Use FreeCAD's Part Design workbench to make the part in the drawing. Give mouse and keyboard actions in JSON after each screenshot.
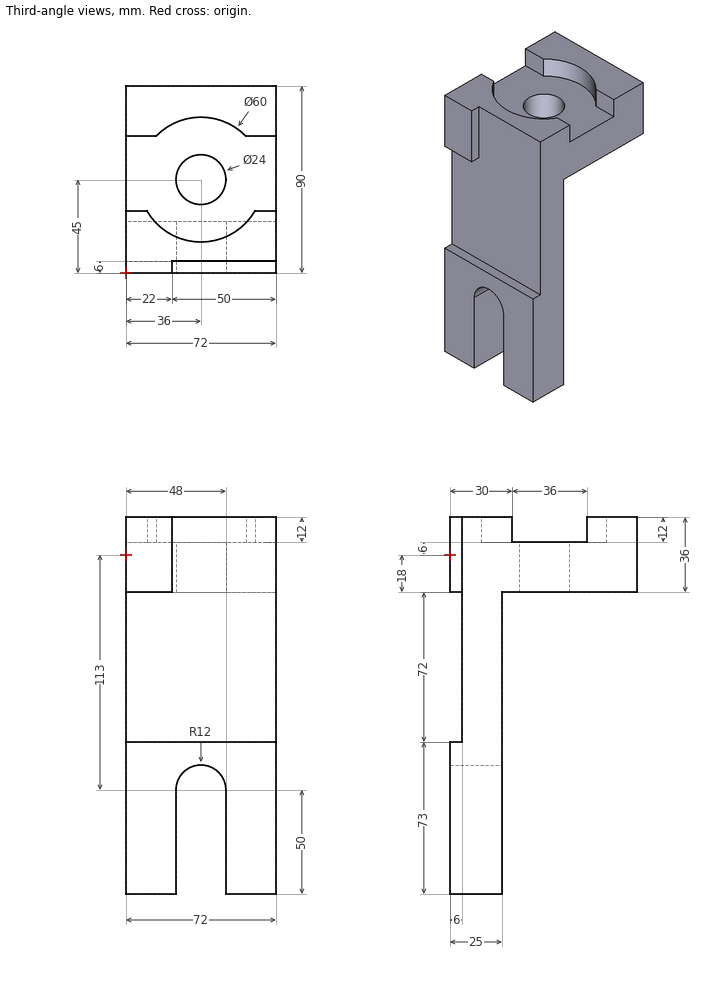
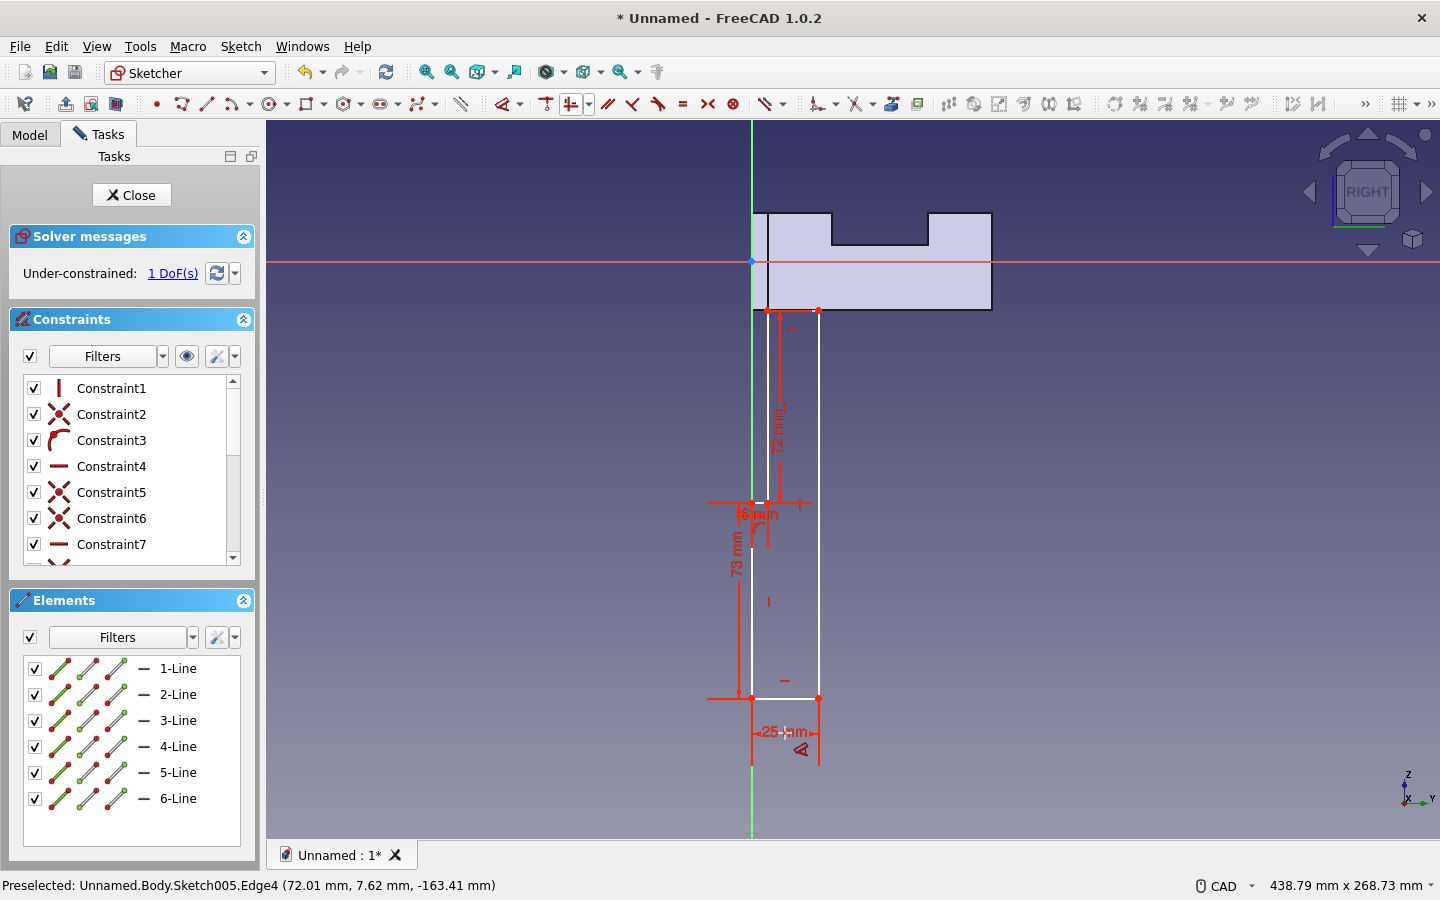
{"action": "left_click", "coordinate": [768, 311]}
{"action": "left_click", "coordinate": [718, 286]}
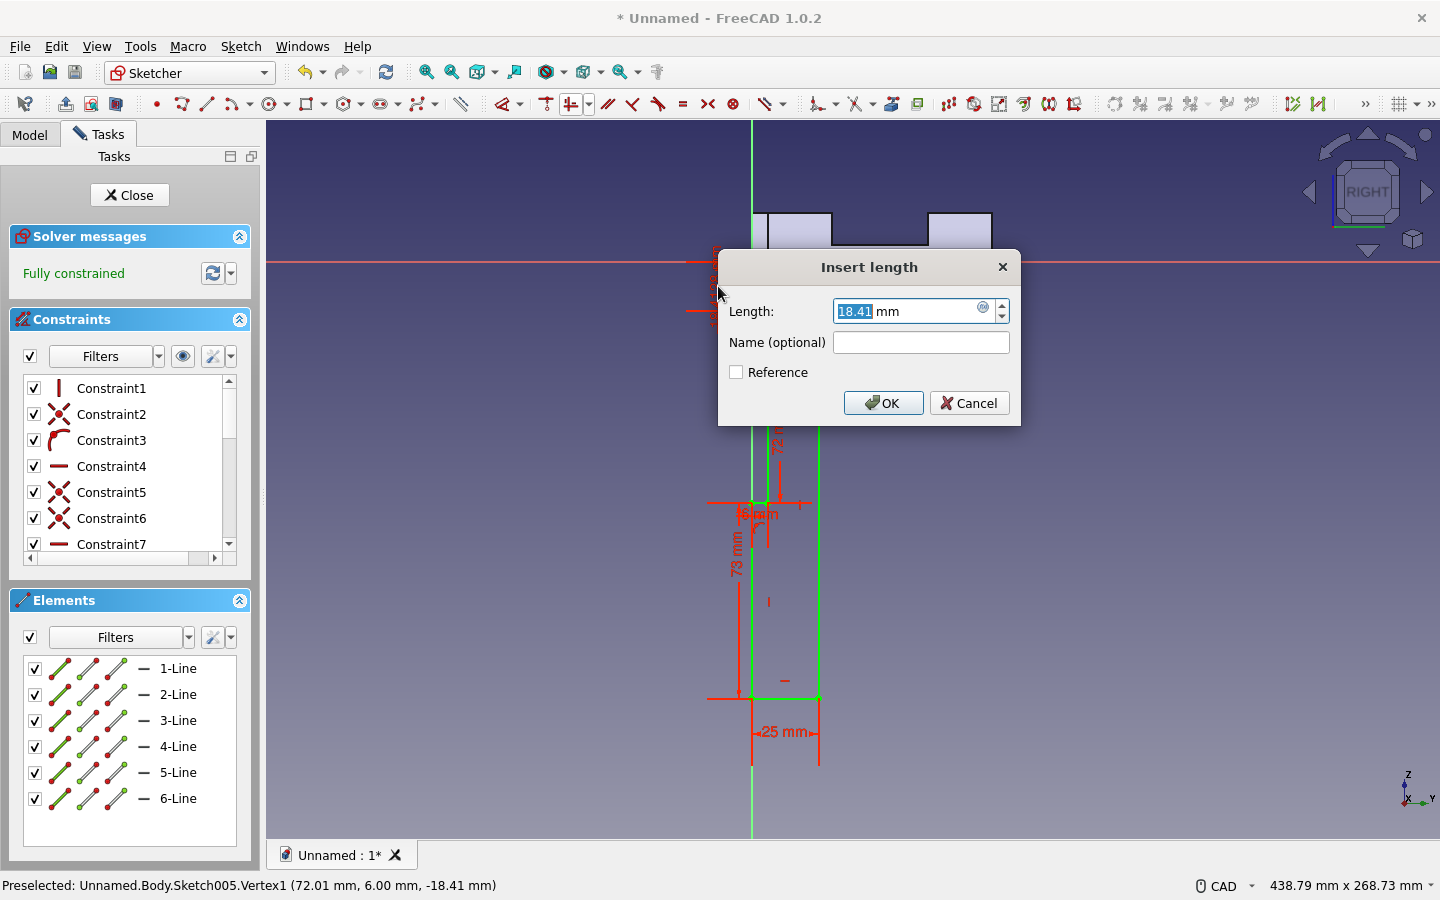
{"action": "type", "text": "18"}
{"action": "key", "text": "Return"}
{"action": "key", "text": "Escape"}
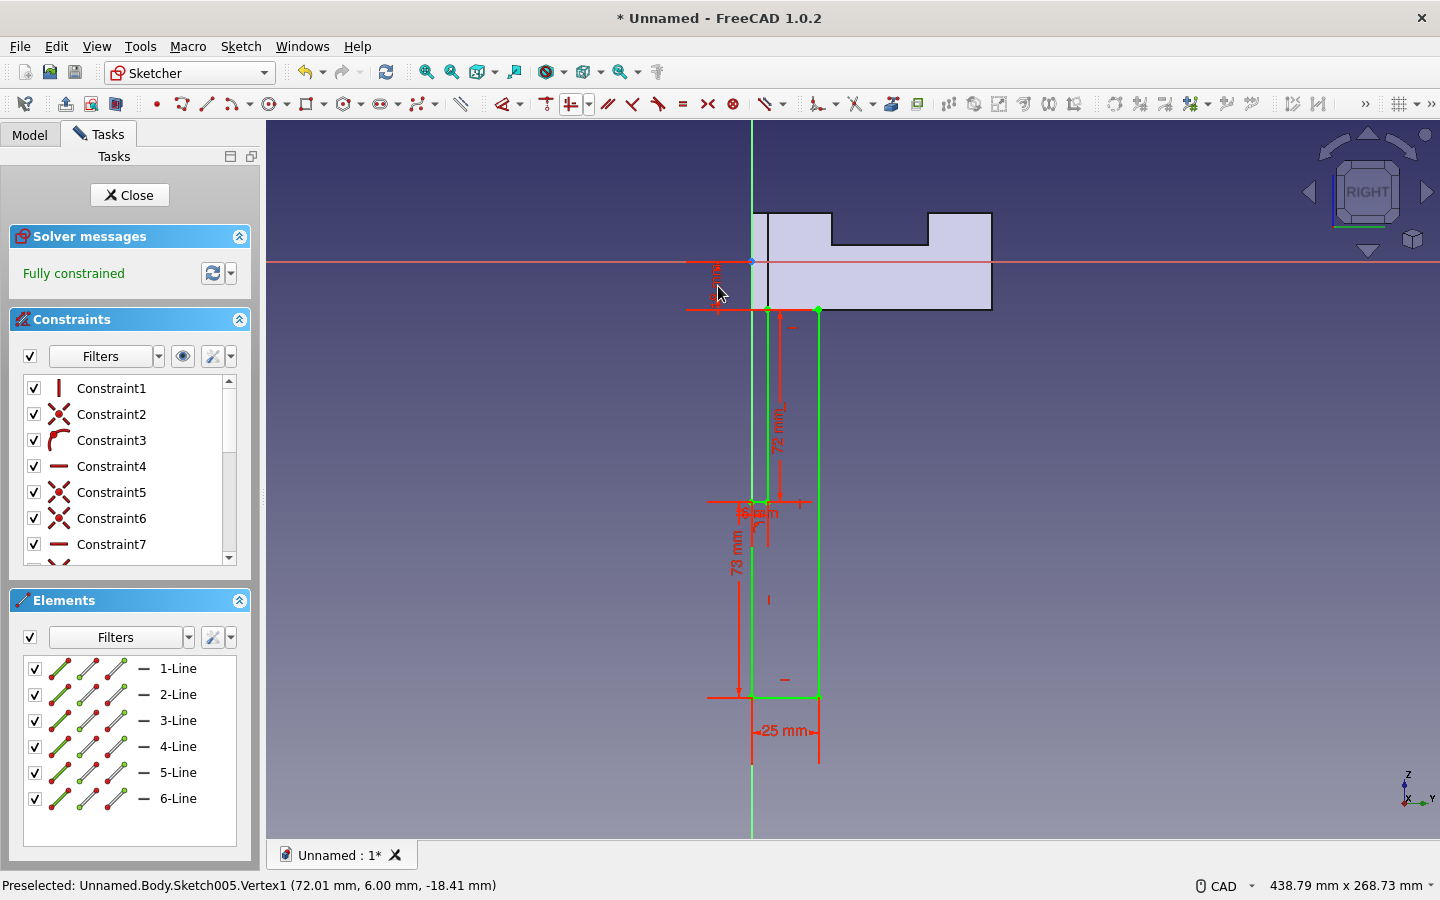
{"action": "left_click", "coordinate": [130, 195]}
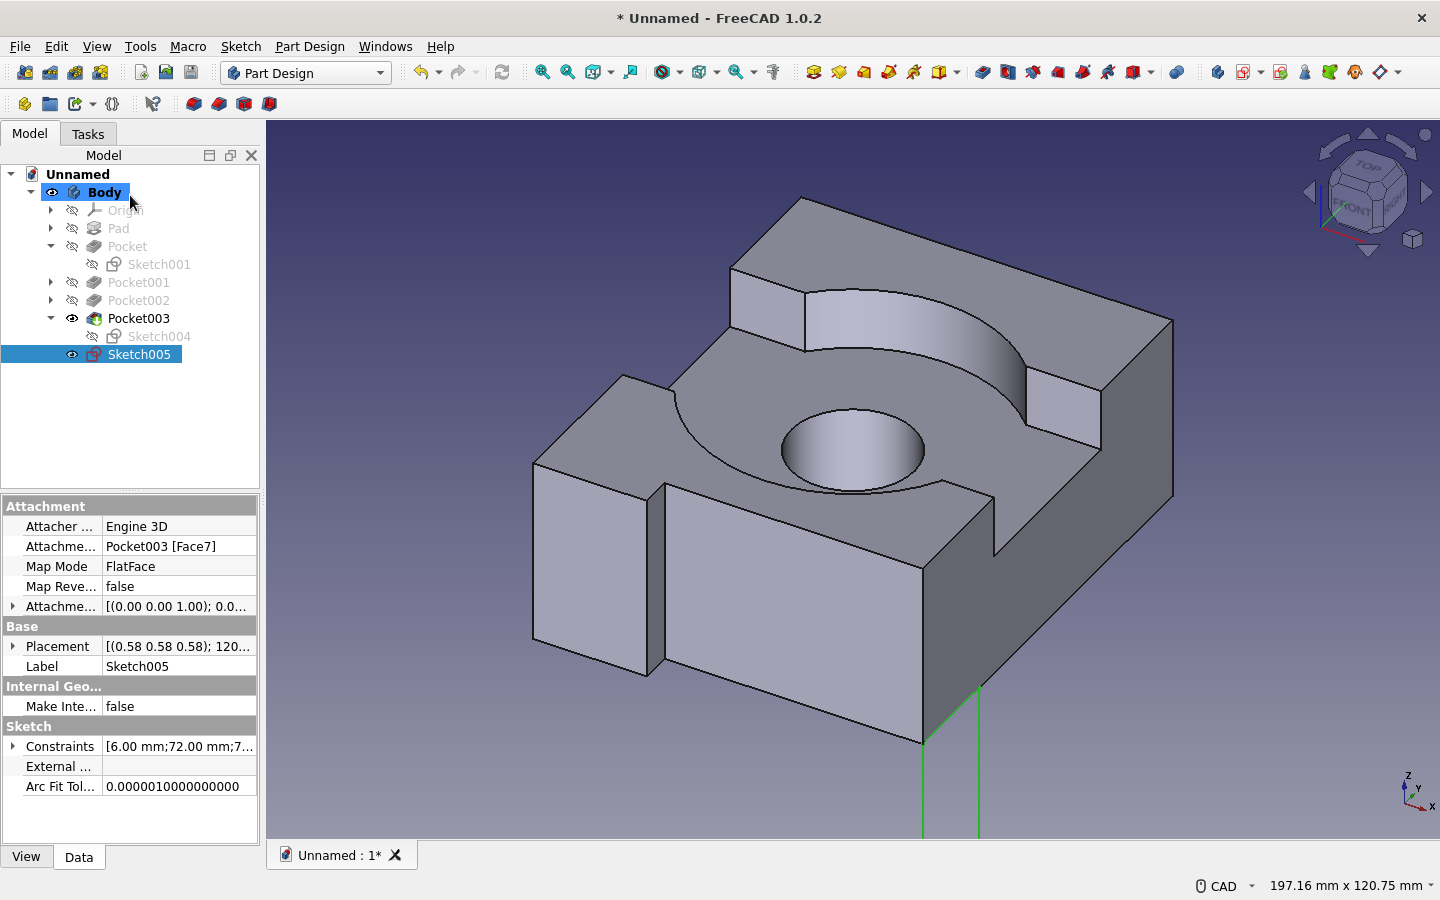
{"action": "left_click", "coordinate": [814, 72]}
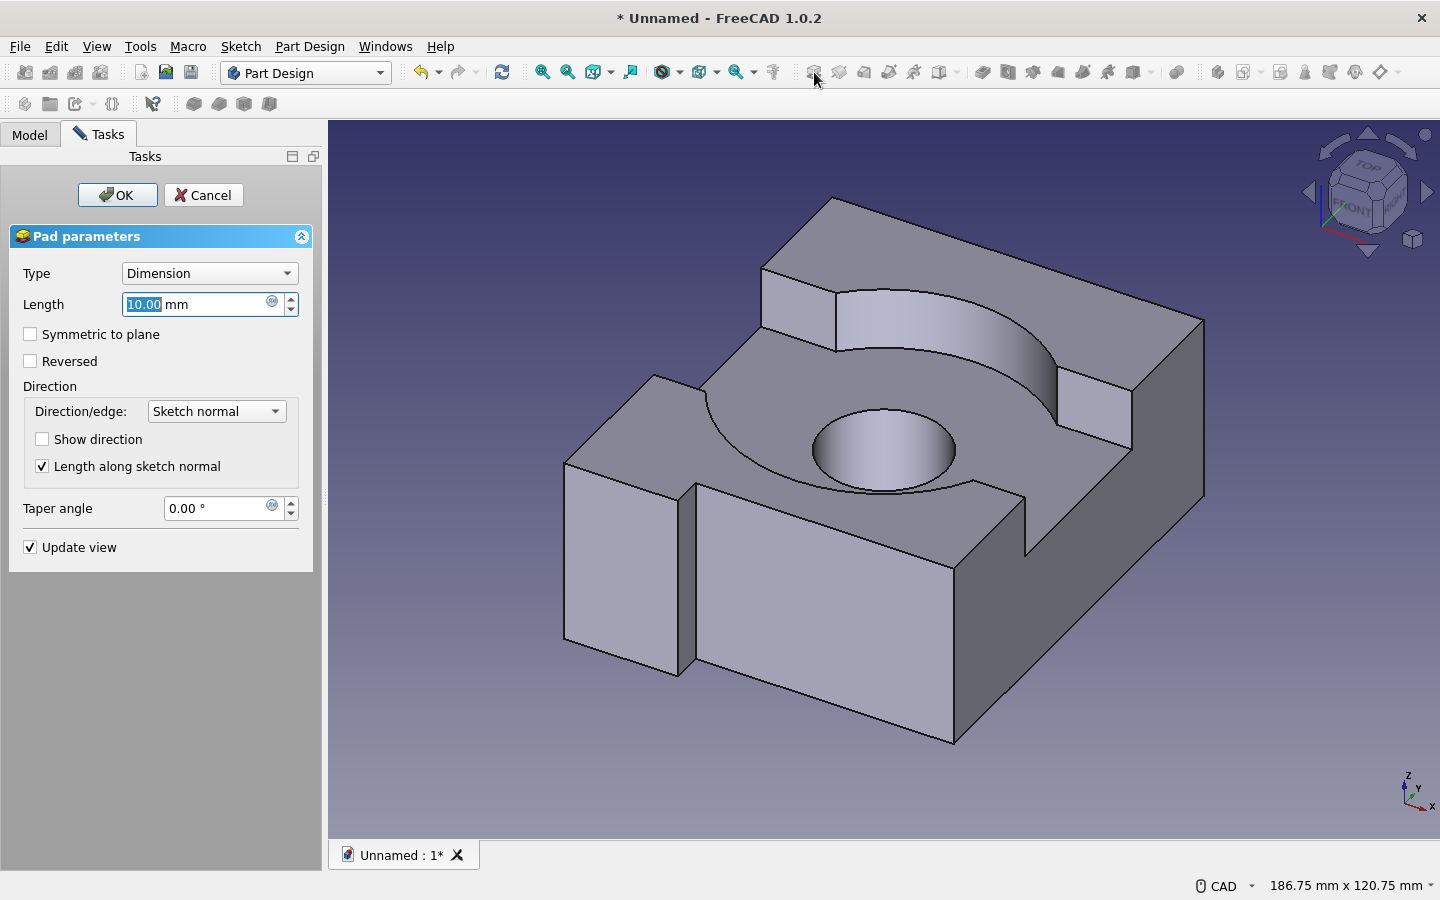
{"action": "type", "text": "72"}
{"action": "key", "text": "Tab"}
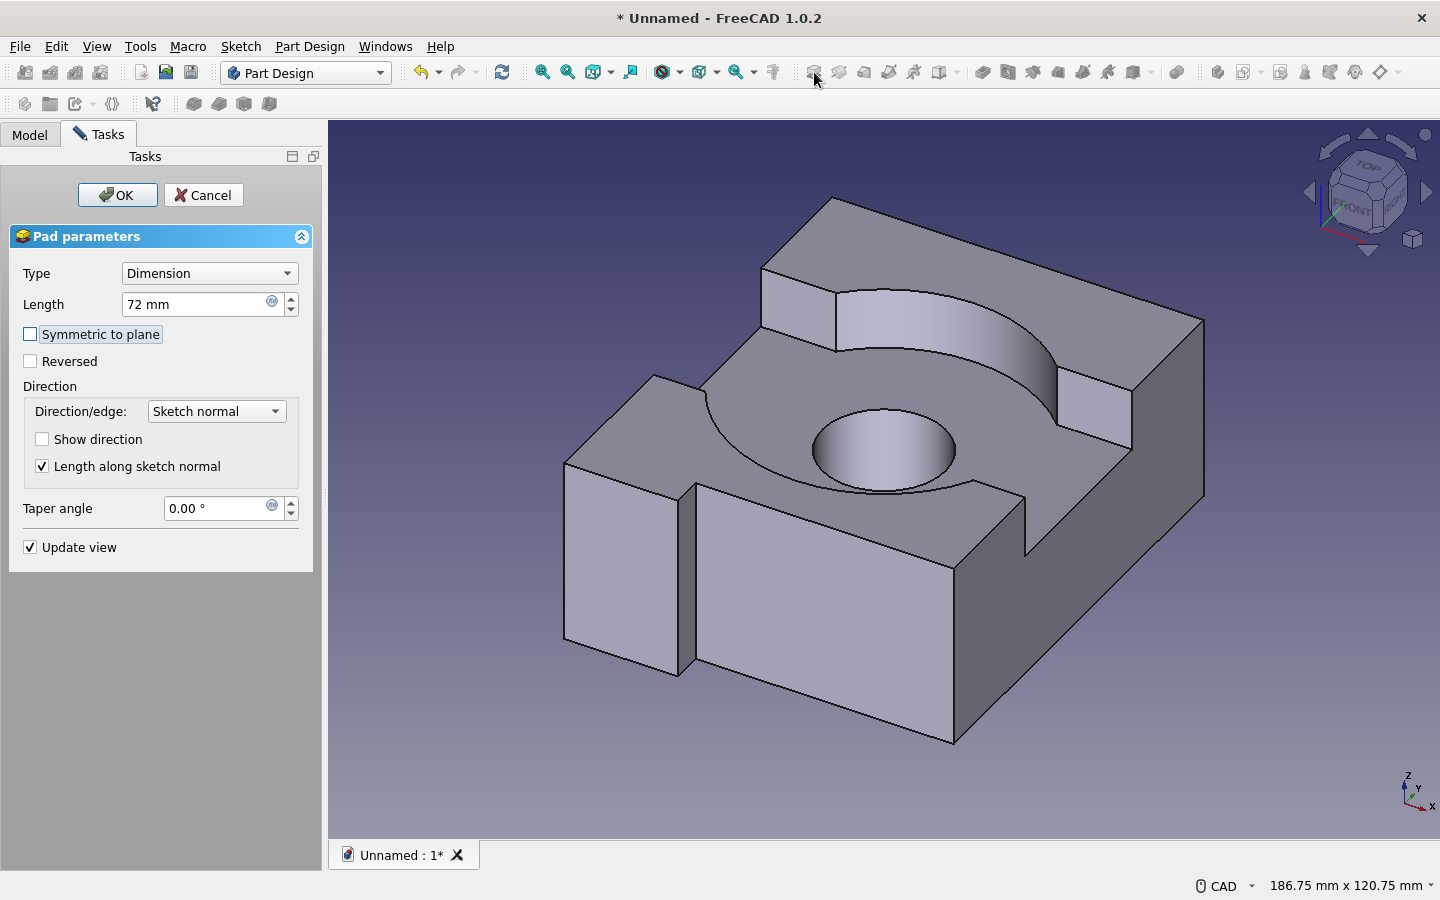
{"action": "left_click", "coordinate": [31, 361]}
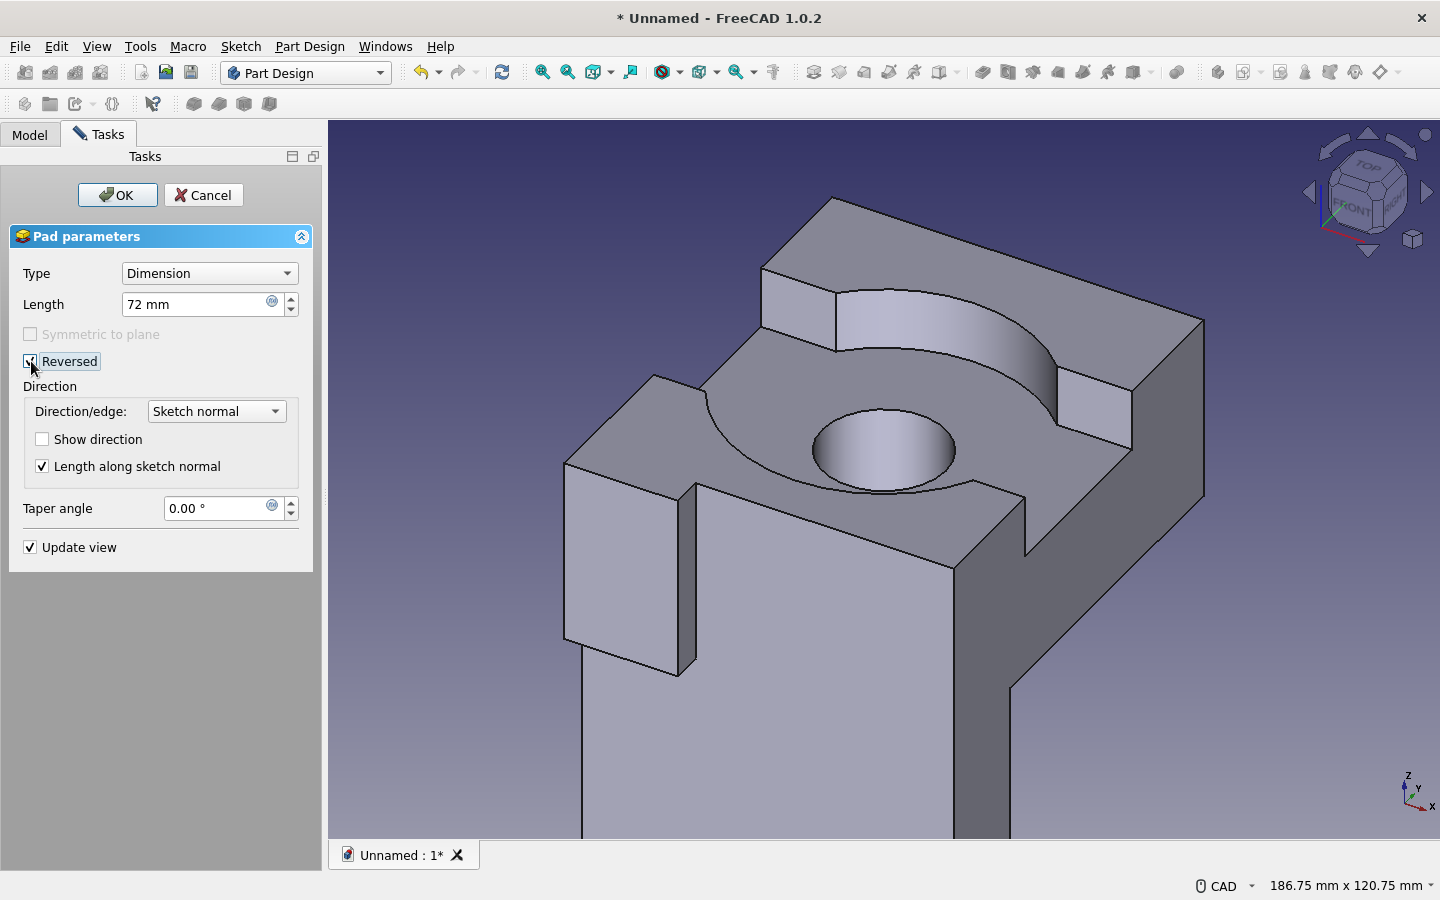
{"action": "left_click", "coordinate": [118, 195]}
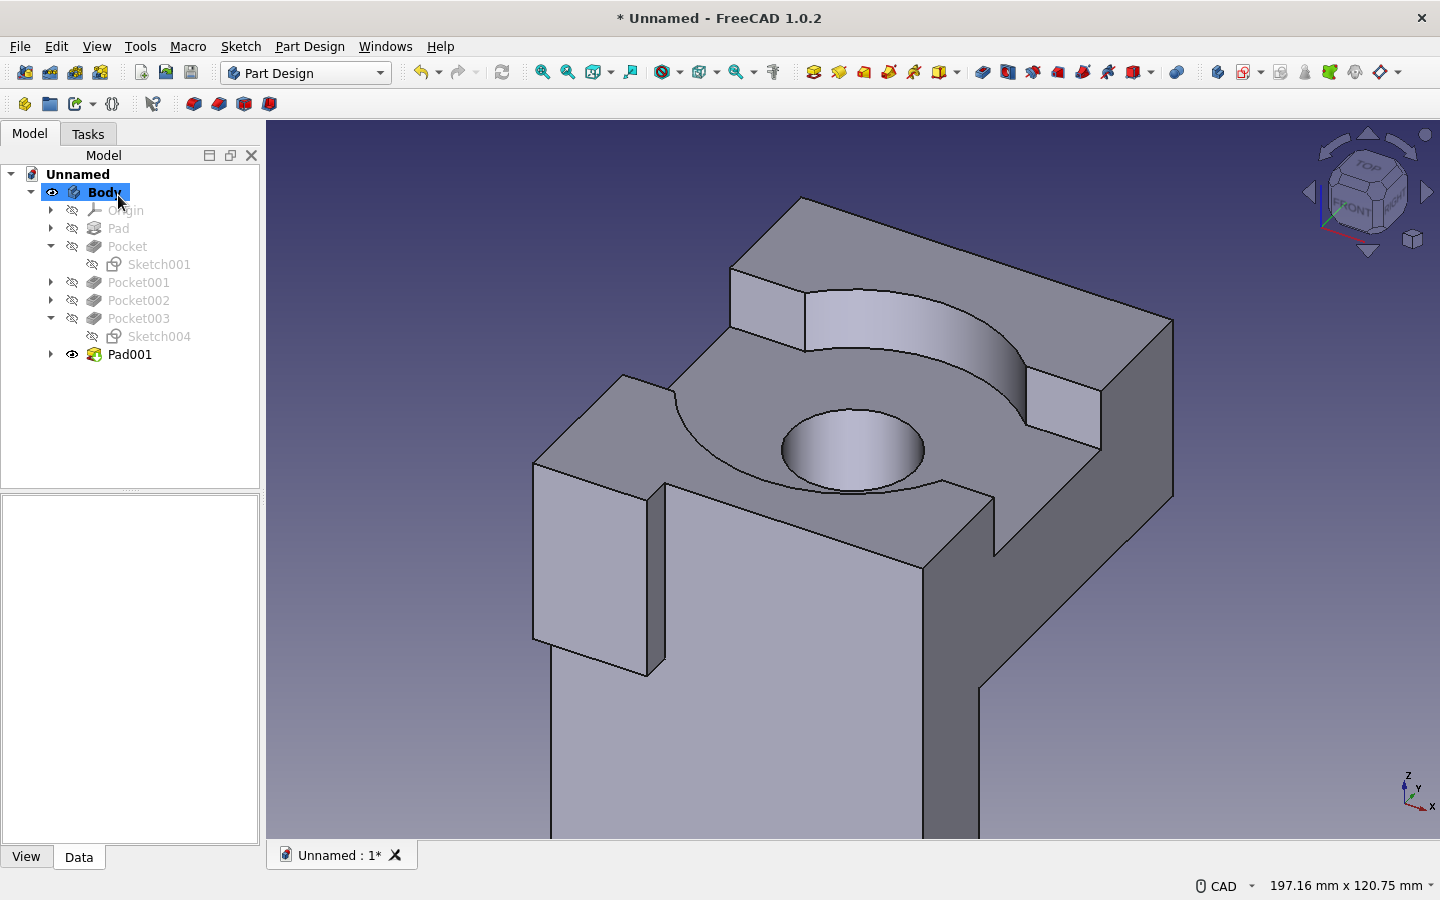
{"action": "key", "text": "v f"}